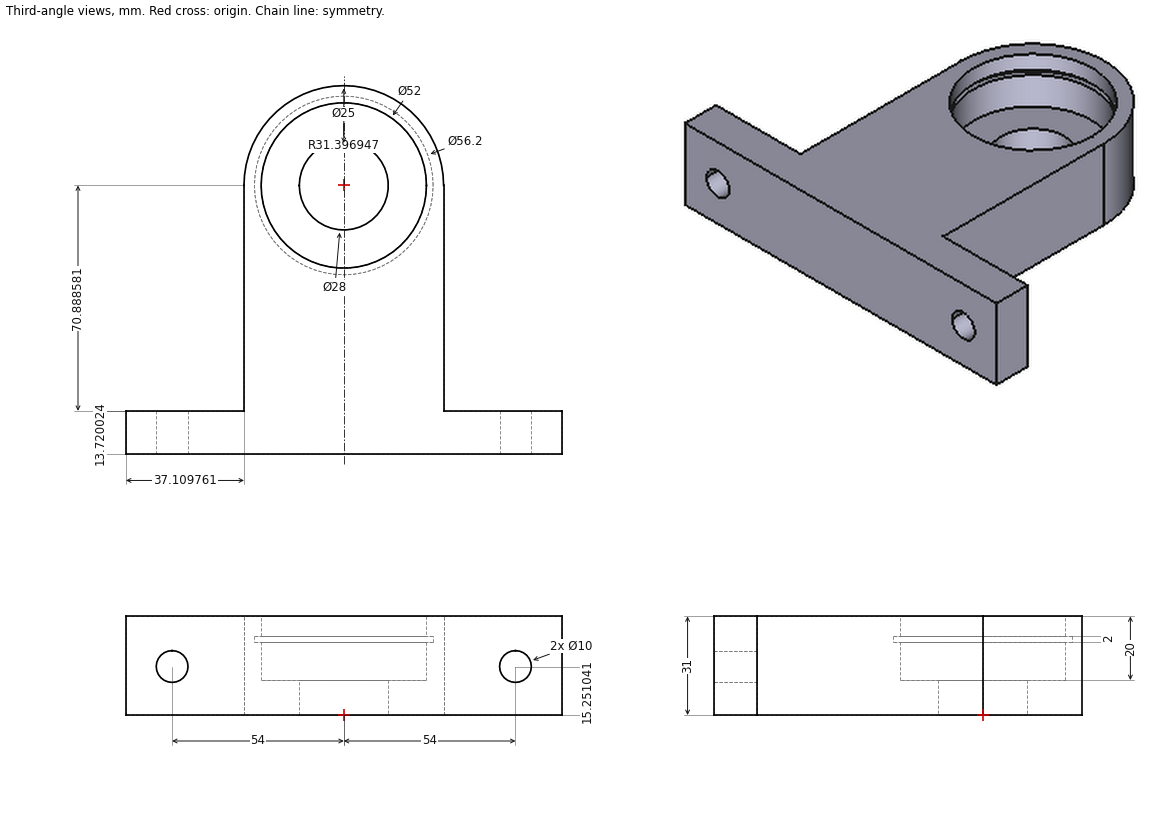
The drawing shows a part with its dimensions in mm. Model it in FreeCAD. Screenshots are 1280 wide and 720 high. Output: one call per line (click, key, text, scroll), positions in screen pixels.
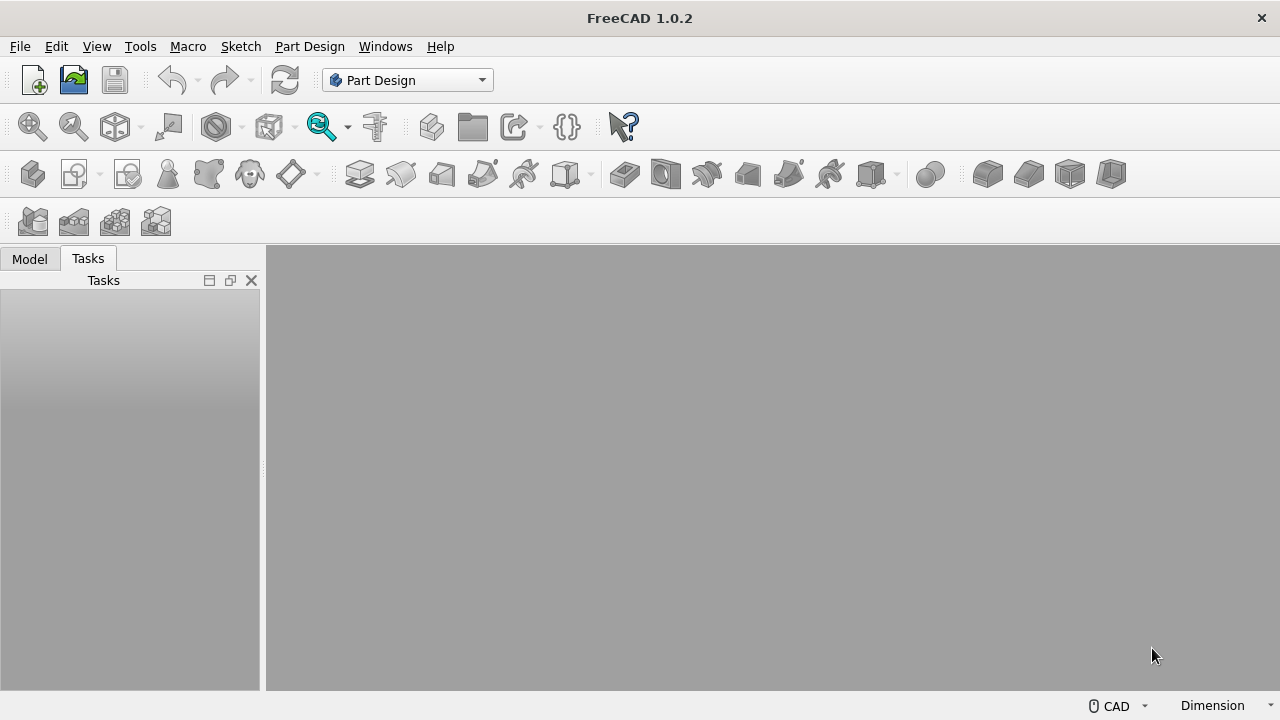
click(33, 80)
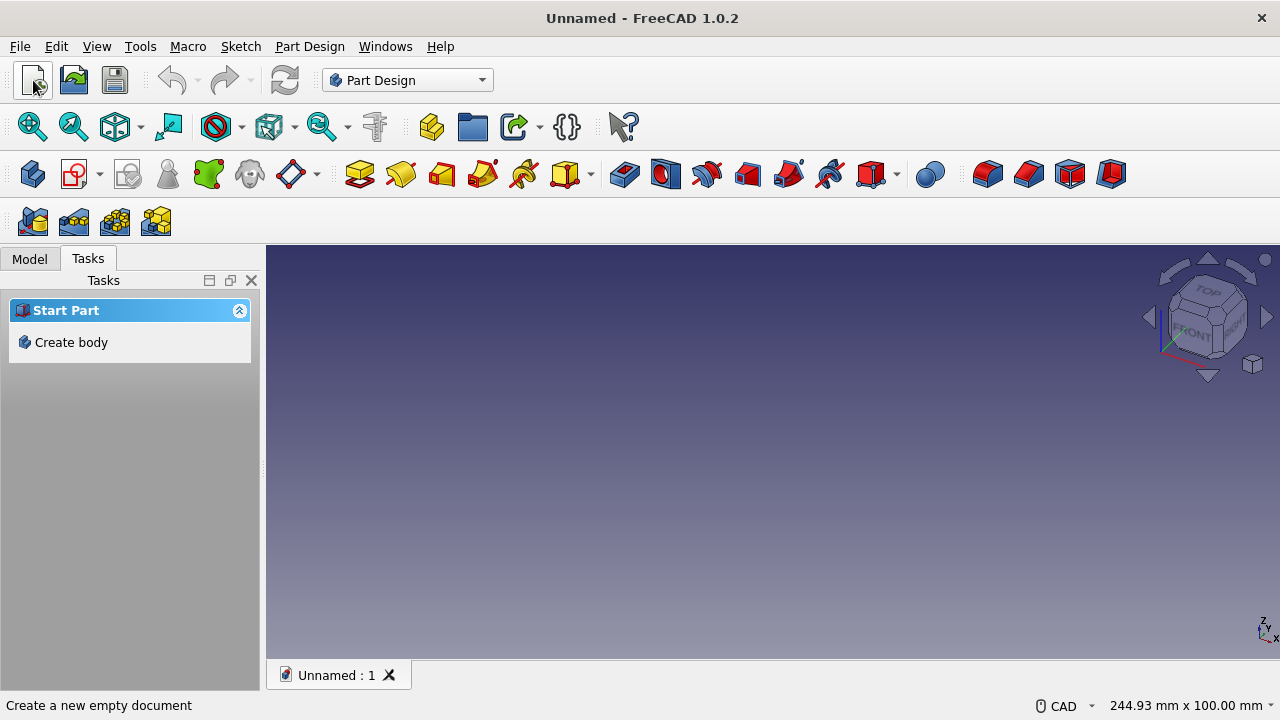
click(74, 174)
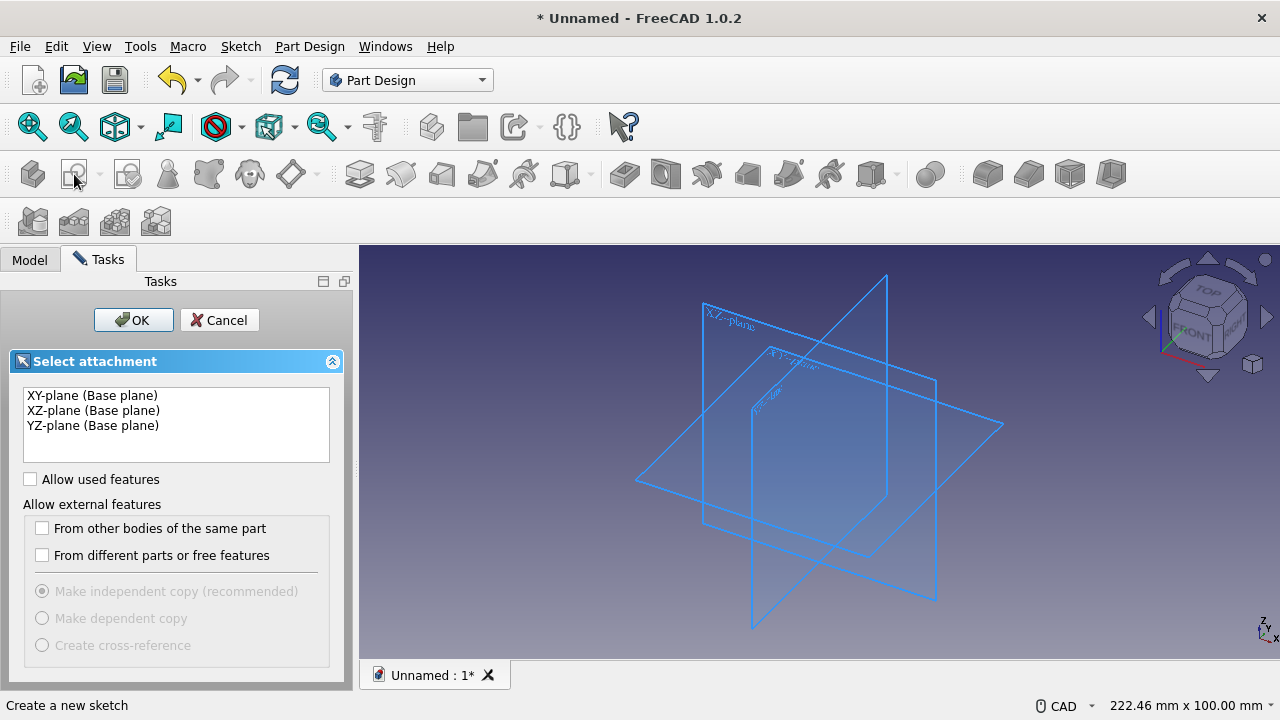
click(84, 396)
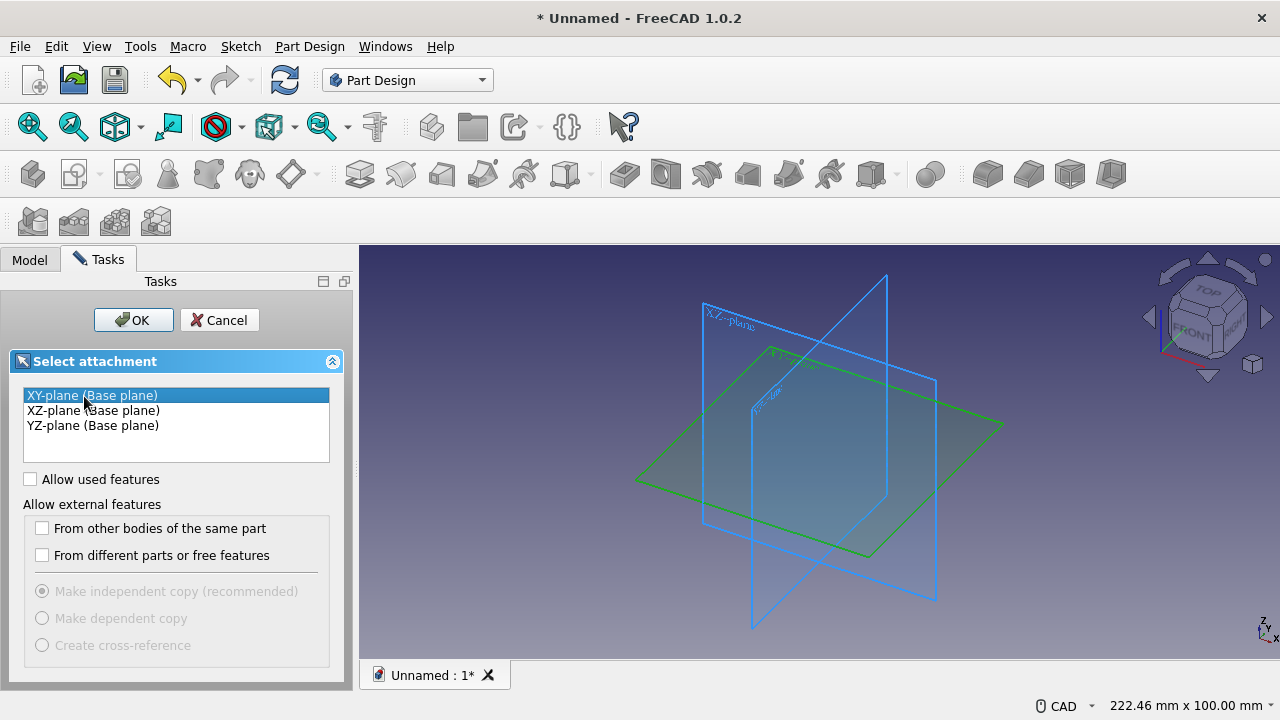
click(134, 320)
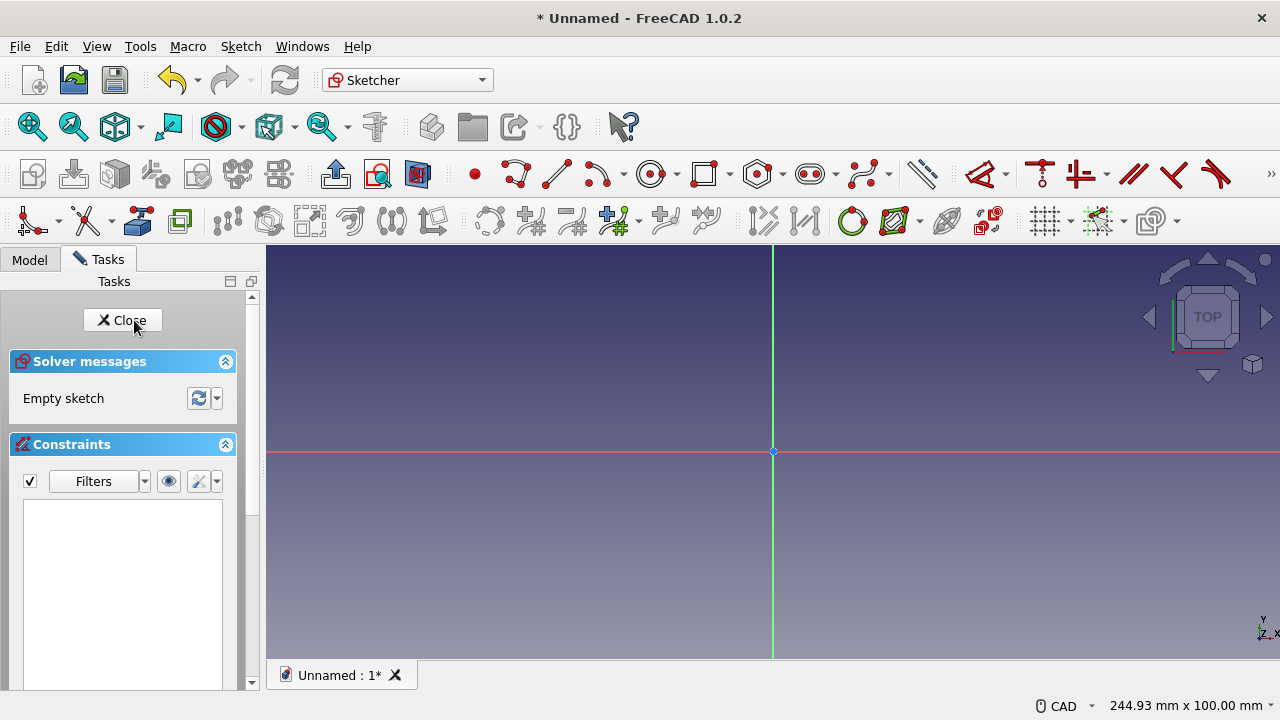
scroll(621, 318, down, 3)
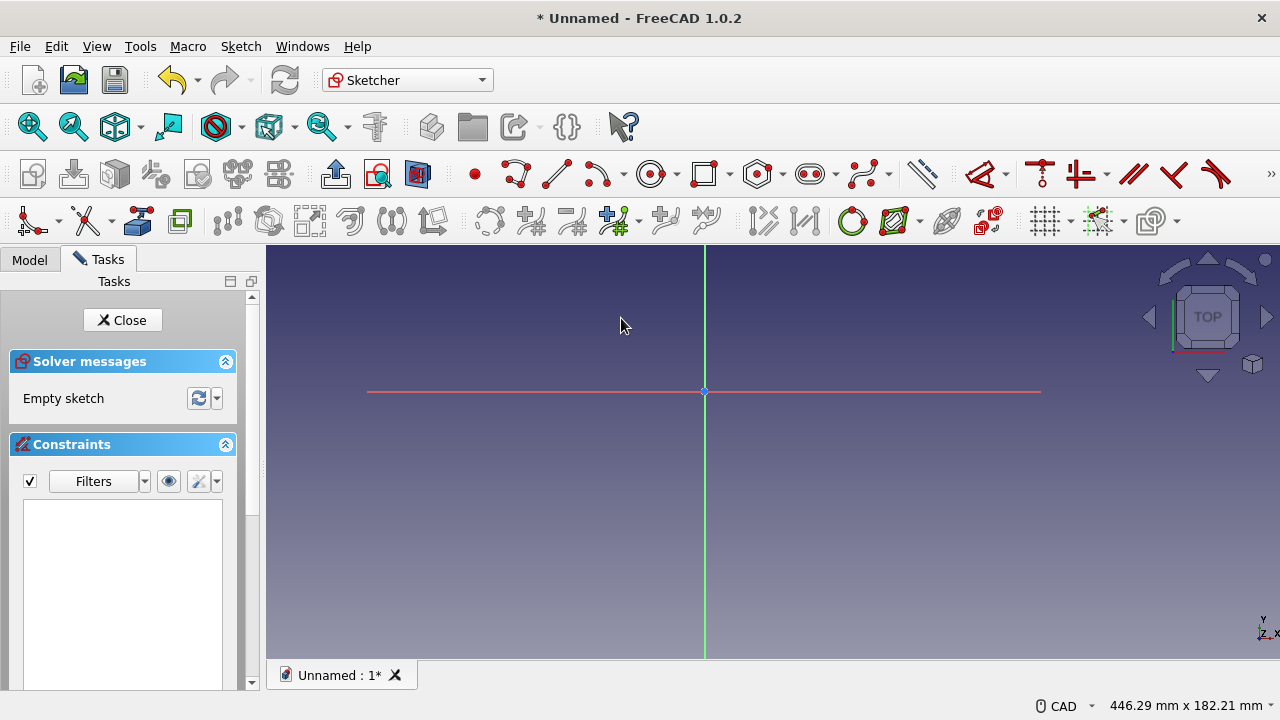
click(516, 174)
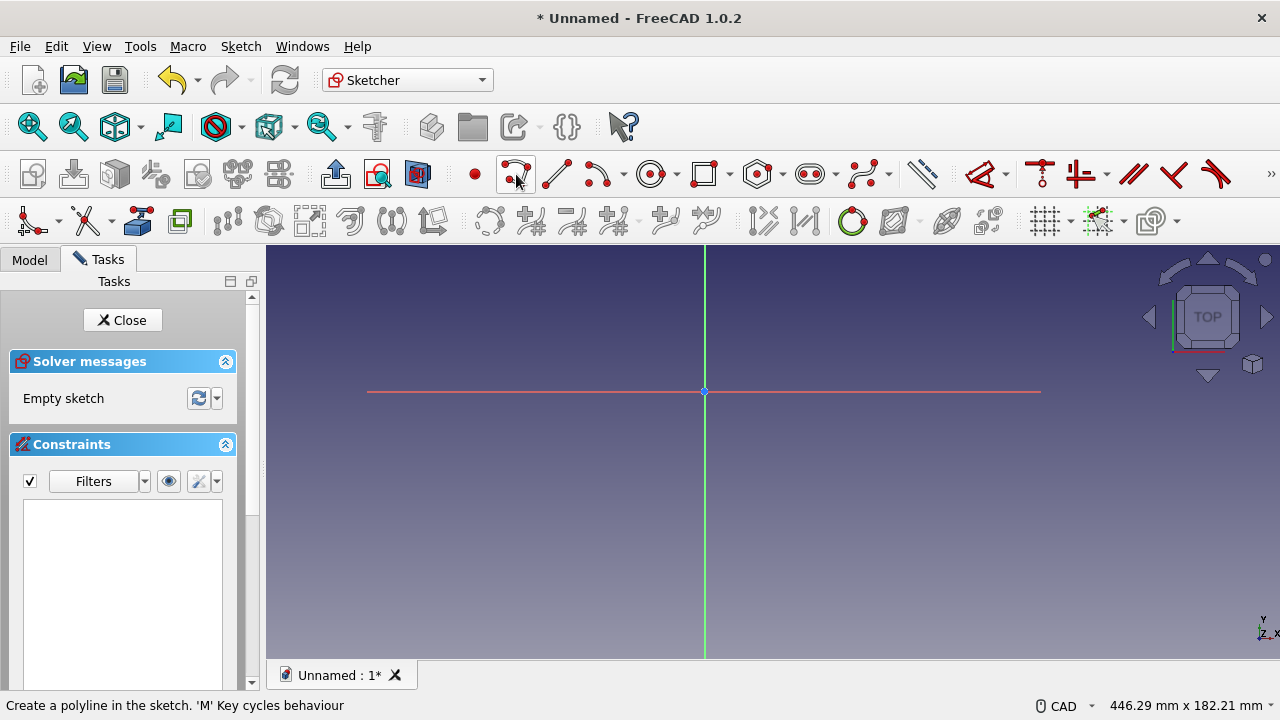
click(633, 392)
click(633, 553)
click(549, 553)
click(549, 584)
click(860, 584)
click(860, 553)
click(776, 553)
click(776, 392)
right_click(776, 392)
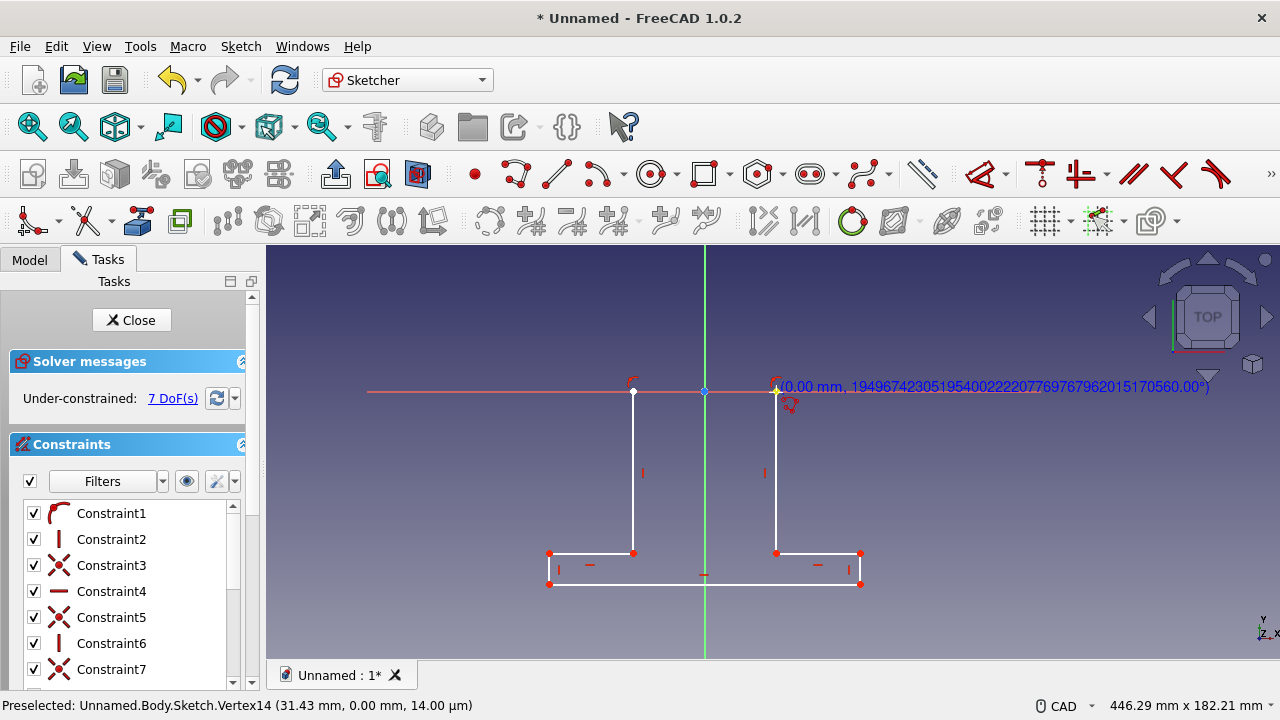
key(g)
key(3)
key(a)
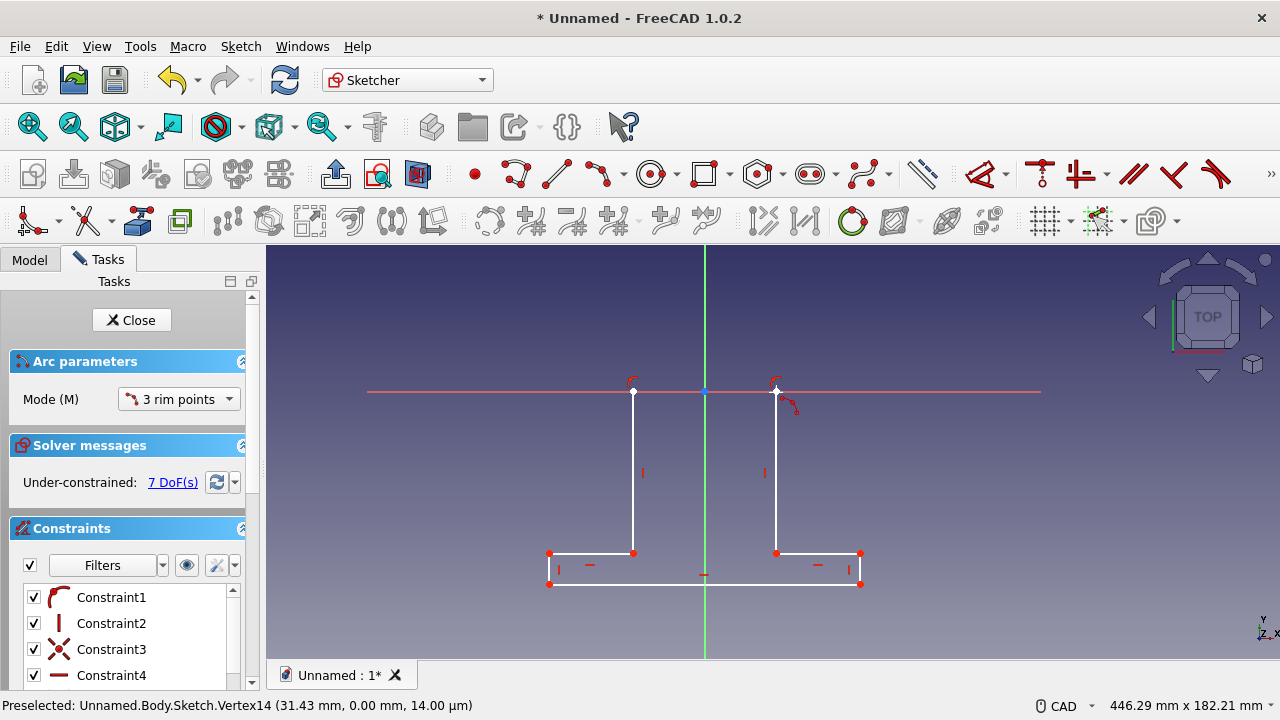
click(776, 392)
click(633, 392)
click(727, 324)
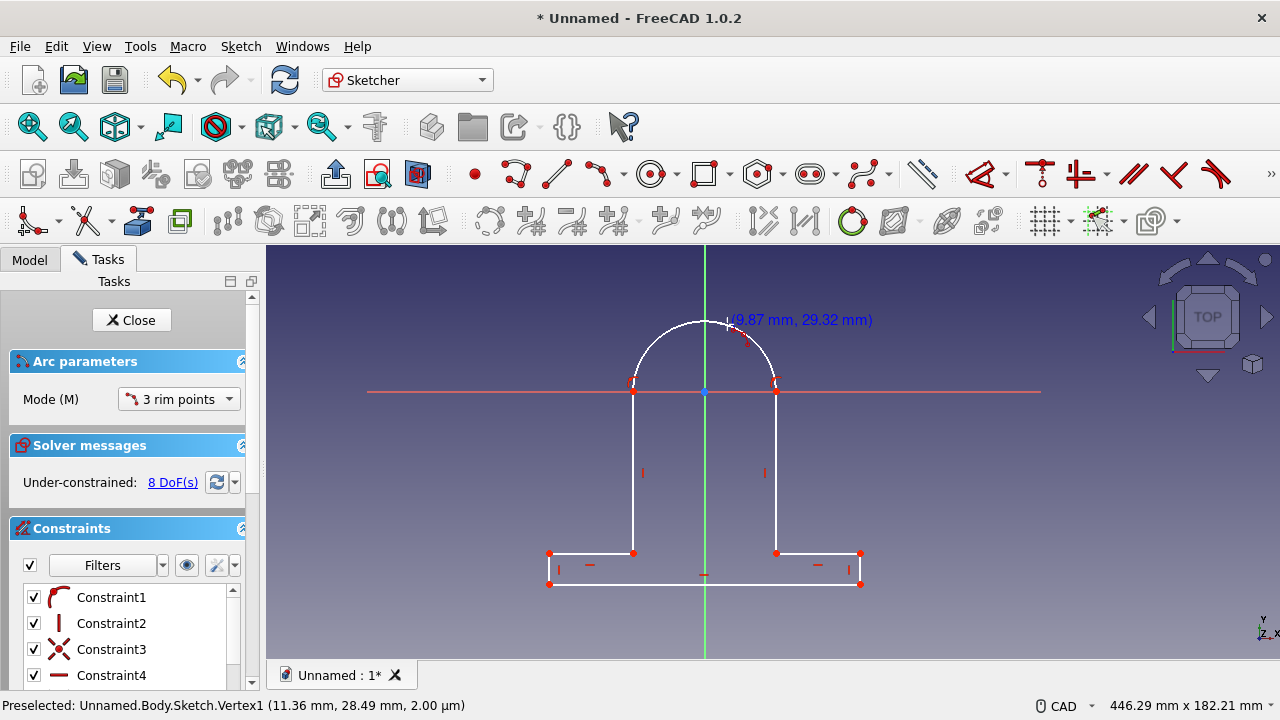
click(650, 174)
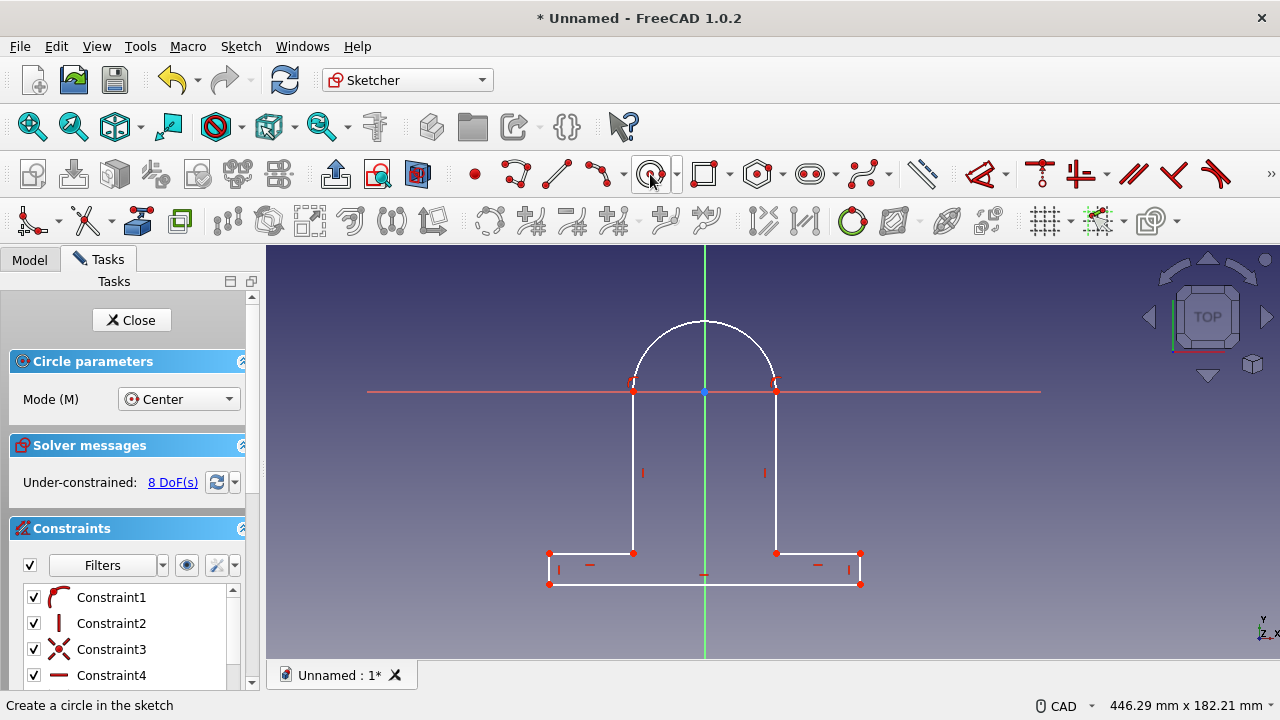
click(705, 392)
click(725, 372)
key(Escape)